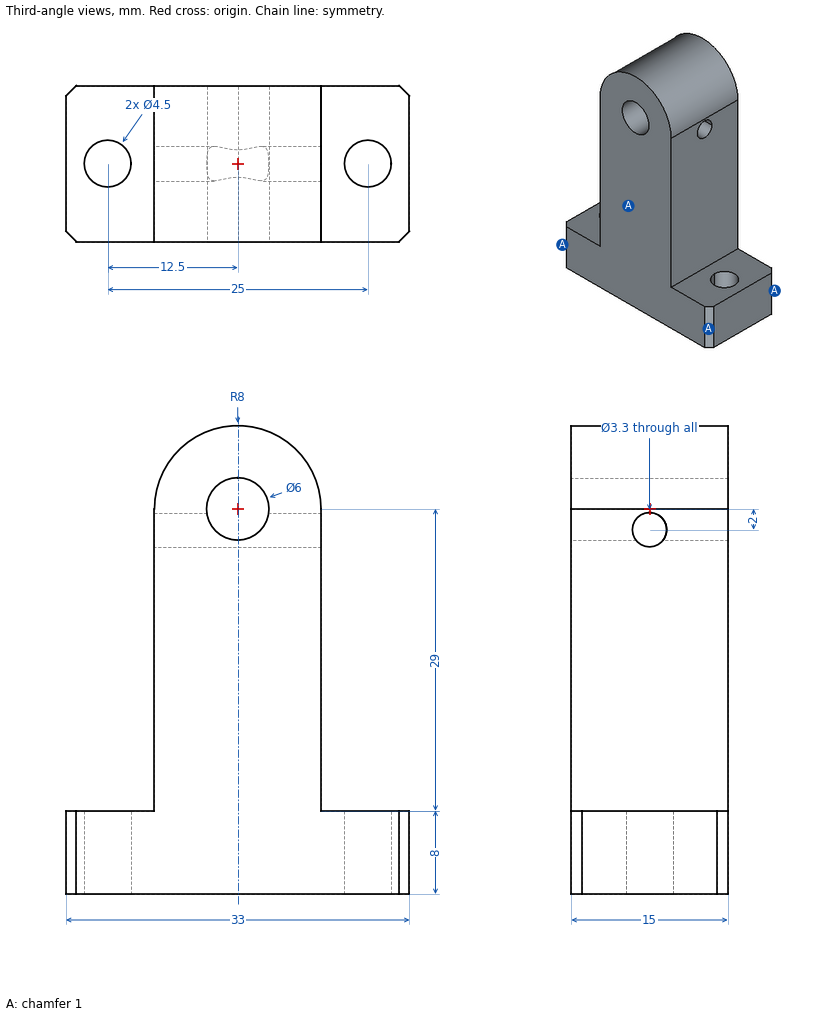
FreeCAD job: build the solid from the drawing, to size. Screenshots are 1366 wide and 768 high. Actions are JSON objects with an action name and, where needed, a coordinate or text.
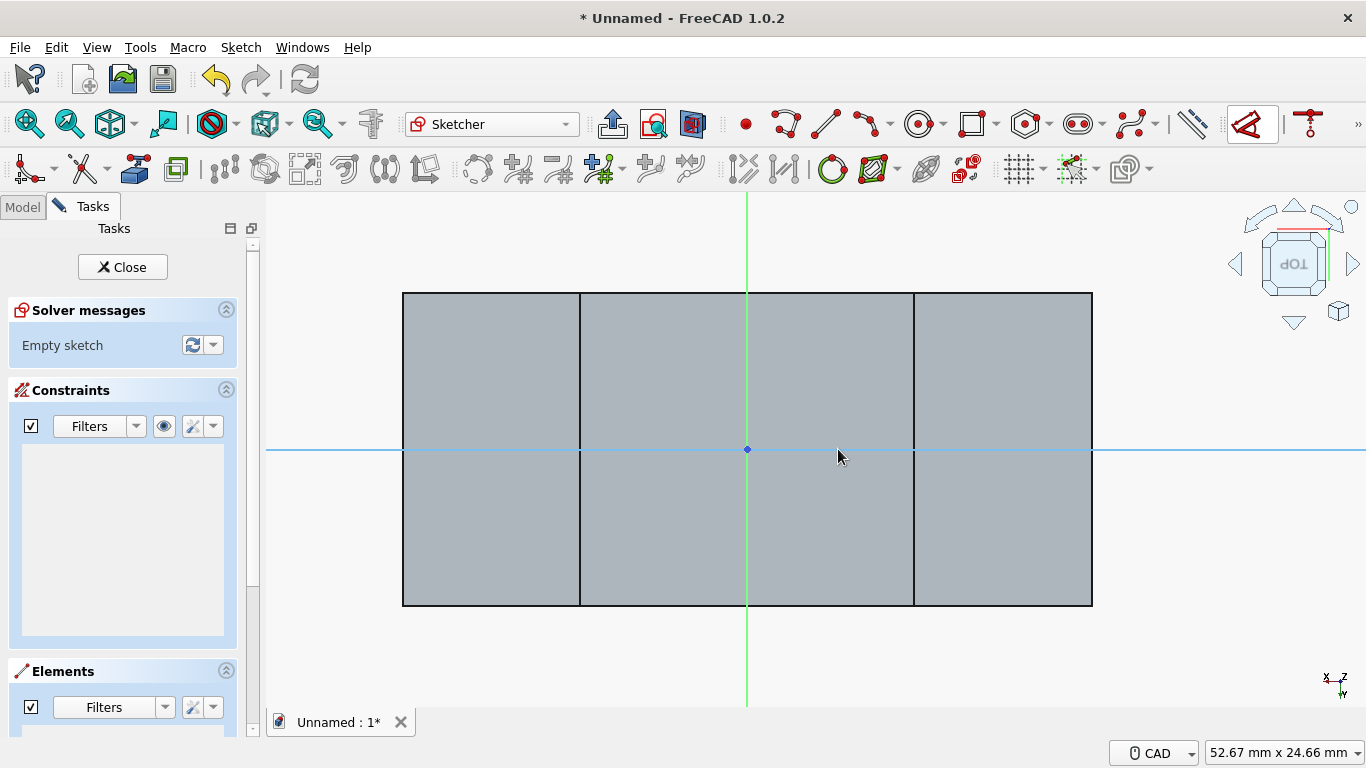
{"action": "key", "text": "g c"}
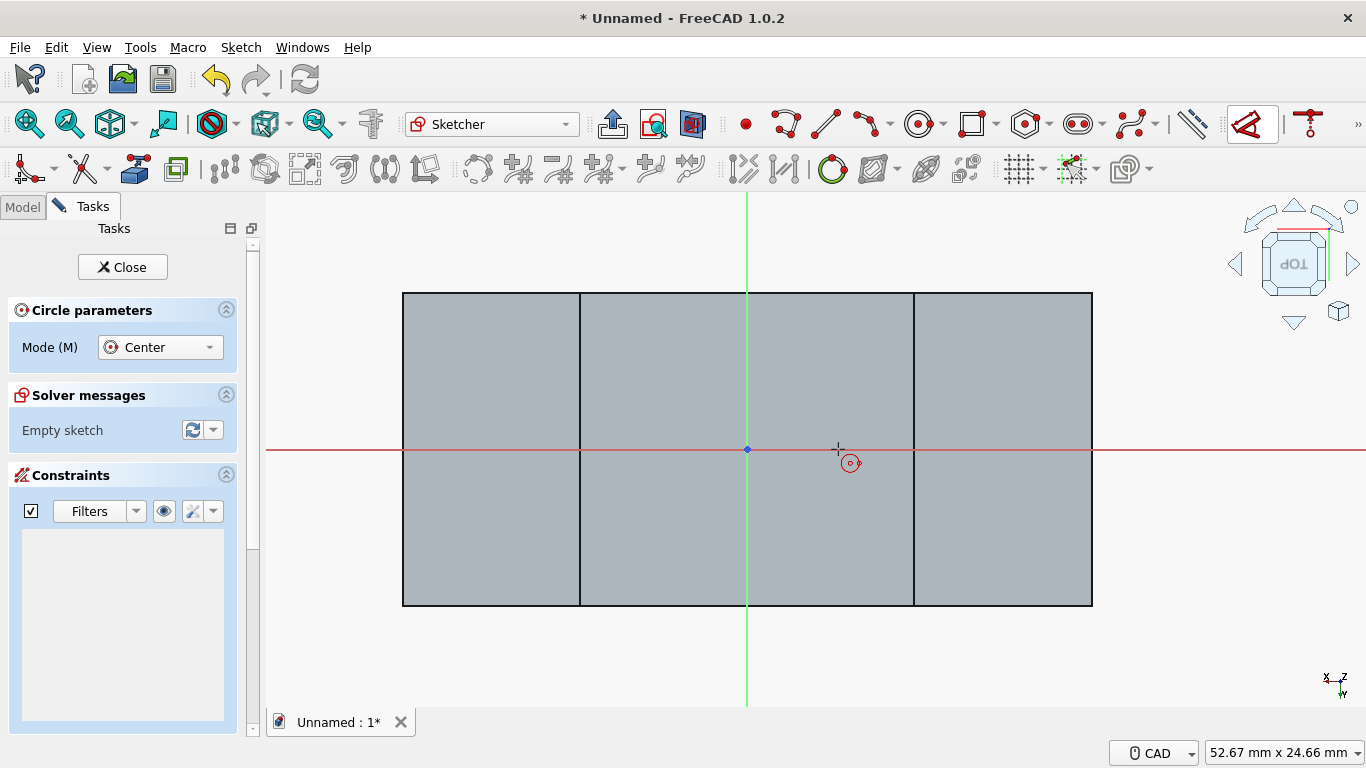
{"action": "left_click", "coordinate": [1008, 449]}
{"action": "mouse_move", "coordinate": [1041, 416]}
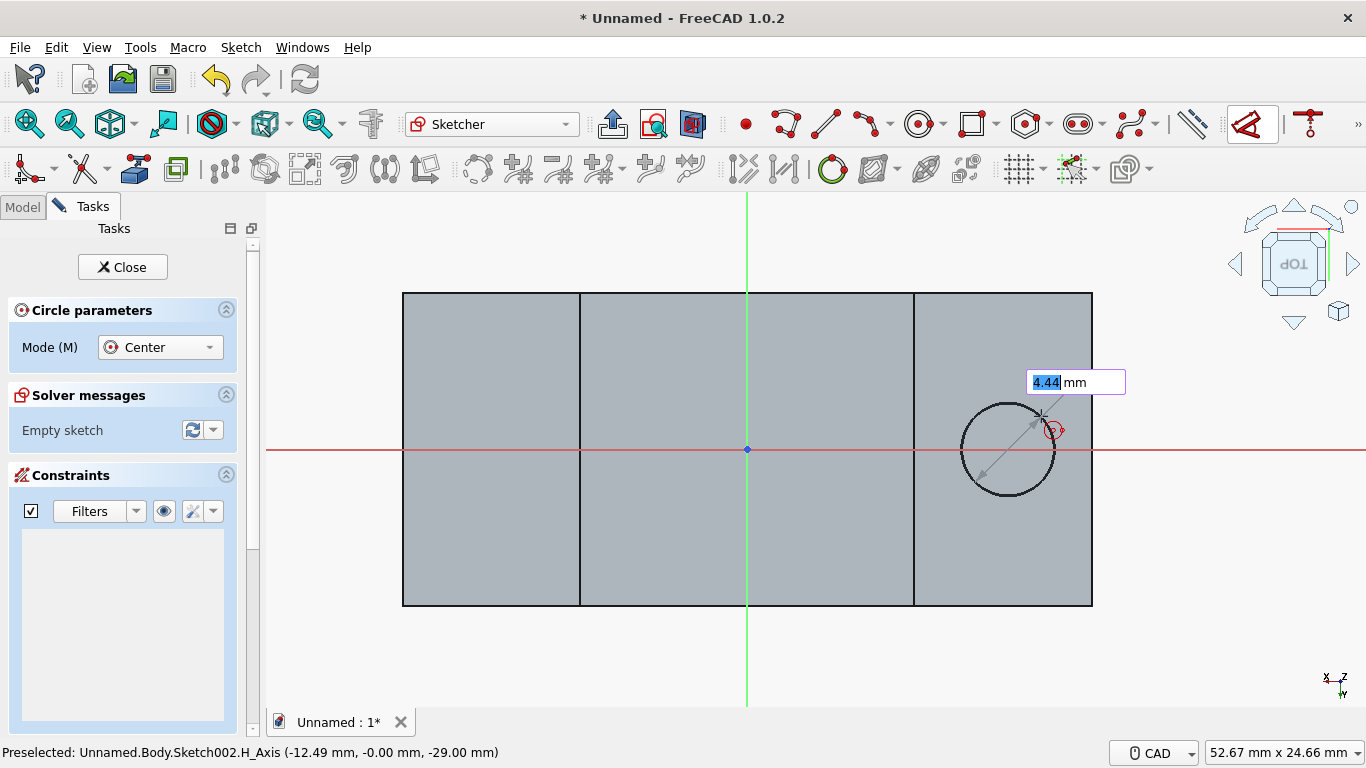
{"action": "type", "text": "4.5"}
{"action": "key", "text": "Return"}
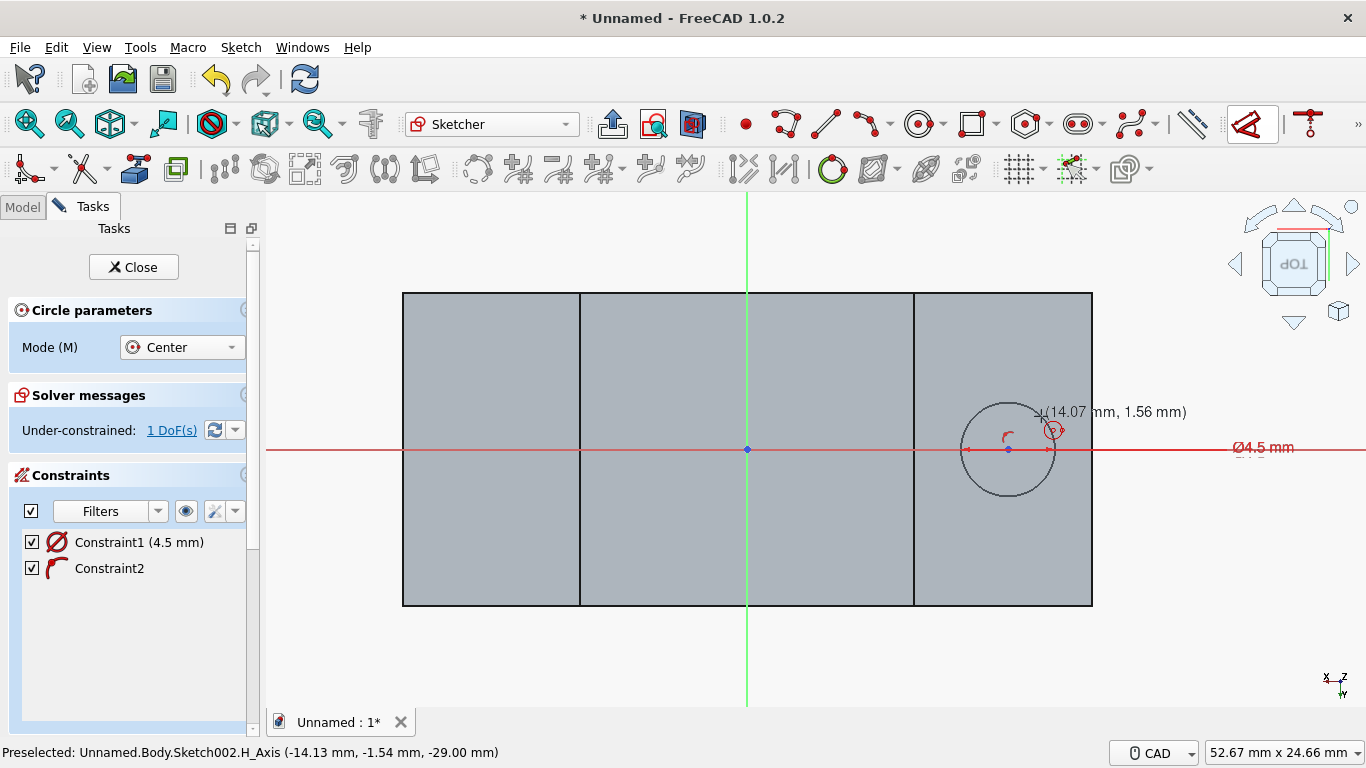
{"action": "left_click", "coordinate": [486, 449]}
{"action": "mouse_move", "coordinate": [519, 416]}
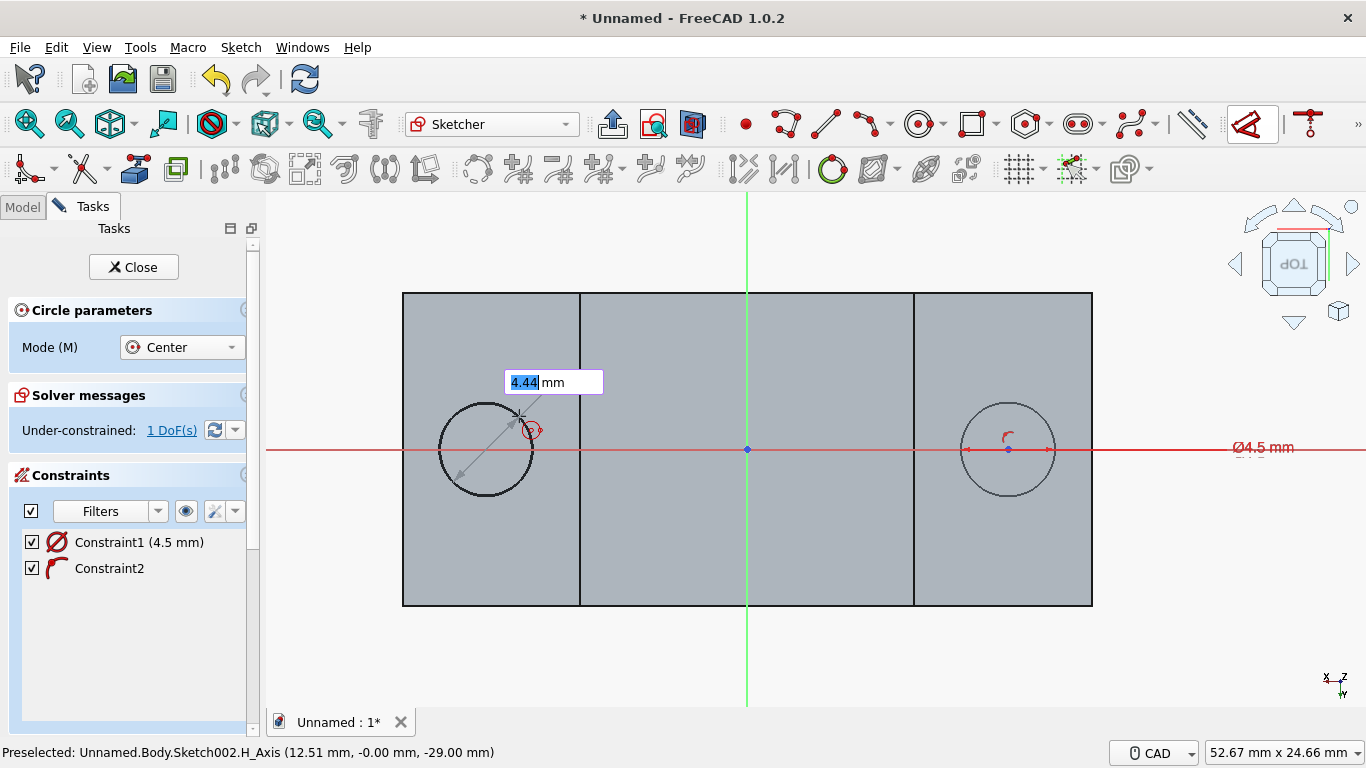
{"action": "type", "text": "4.5"}
{"action": "key", "text": "Return"}
{"action": "key", "text": "Escape"}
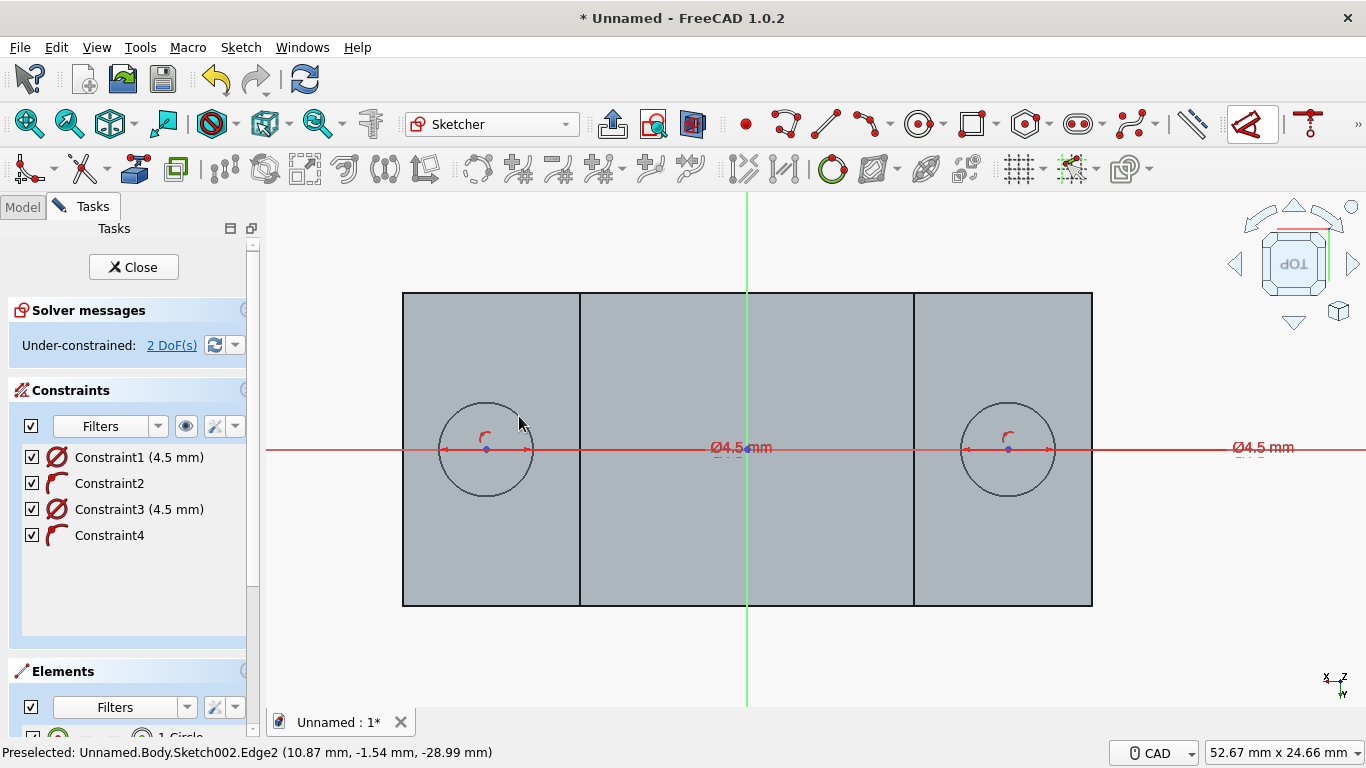
{"action": "left_click", "coordinate": [1246, 124]}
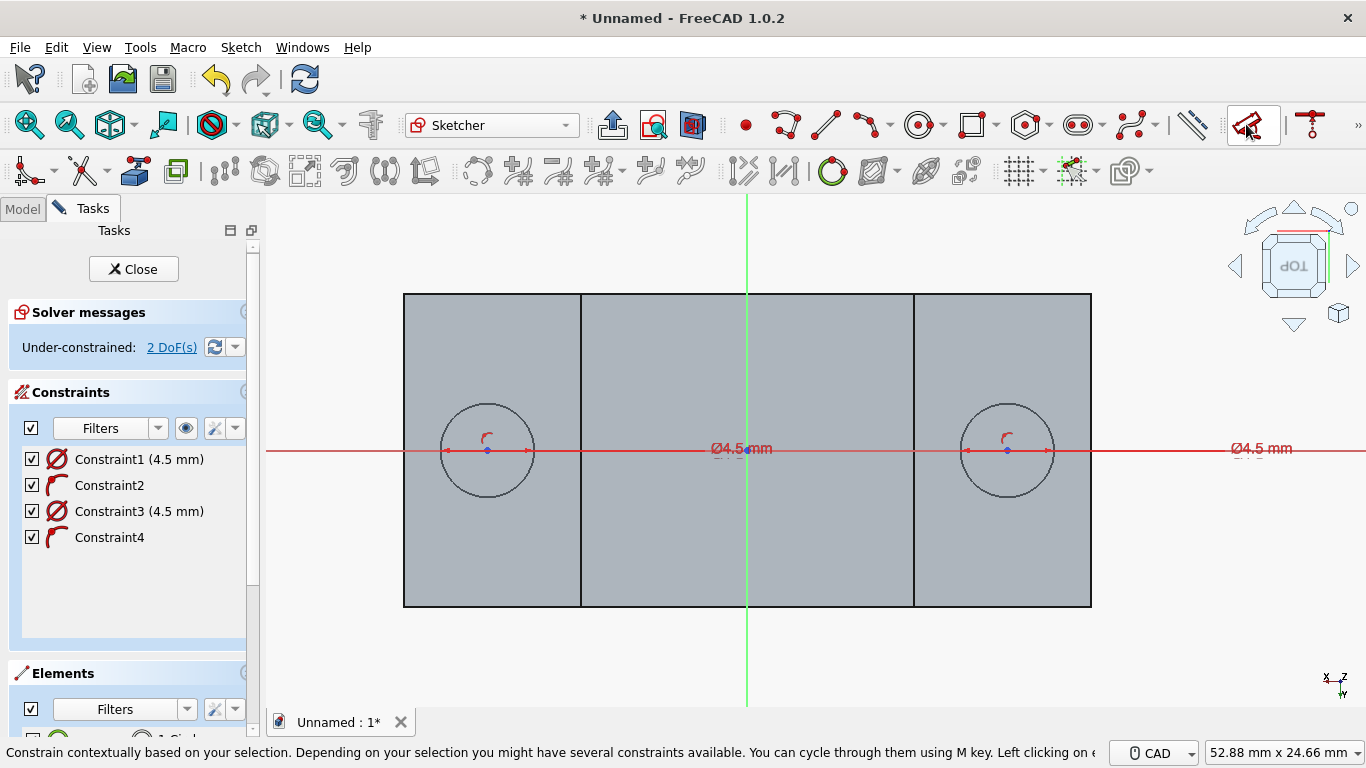
{"action": "left_click", "coordinate": [1007, 450]}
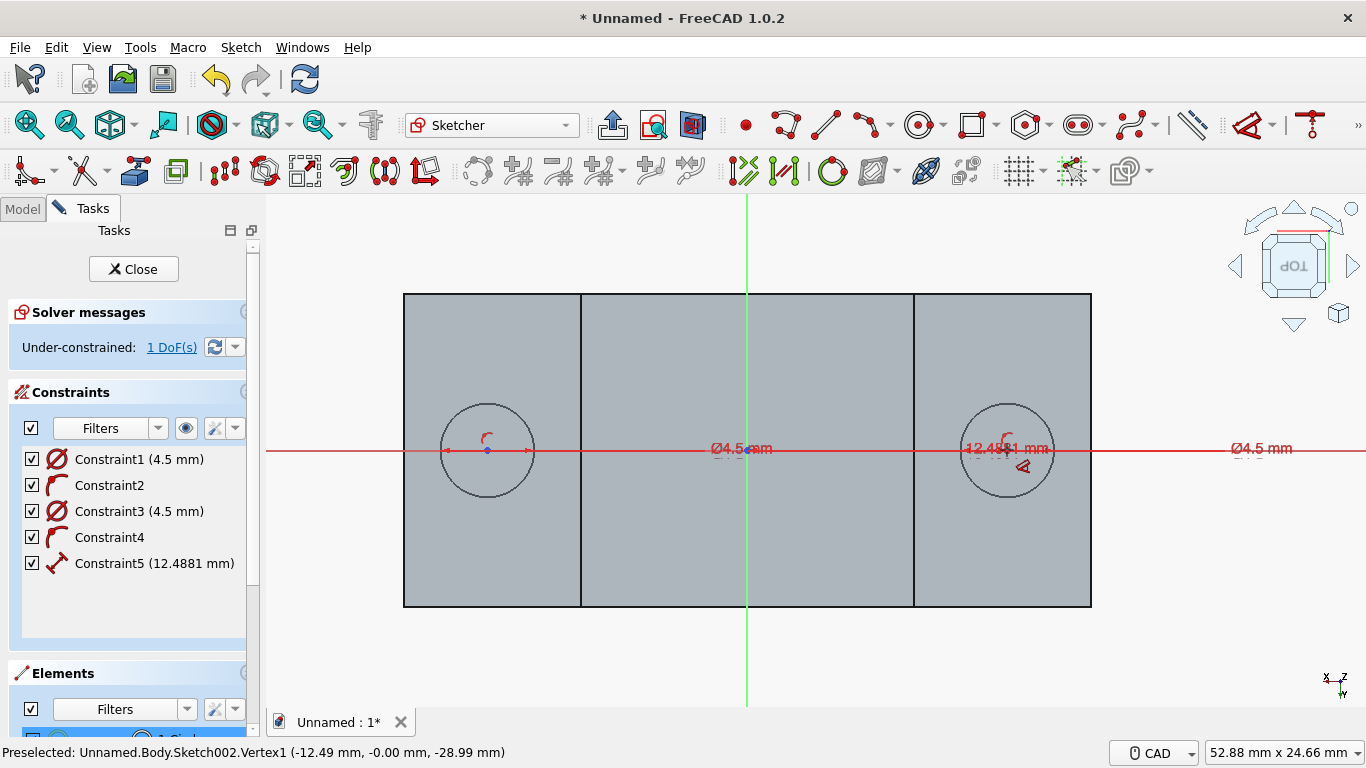
{"action": "left_click", "coordinate": [487, 450]}
{"action": "left_click", "coordinate": [628, 484]}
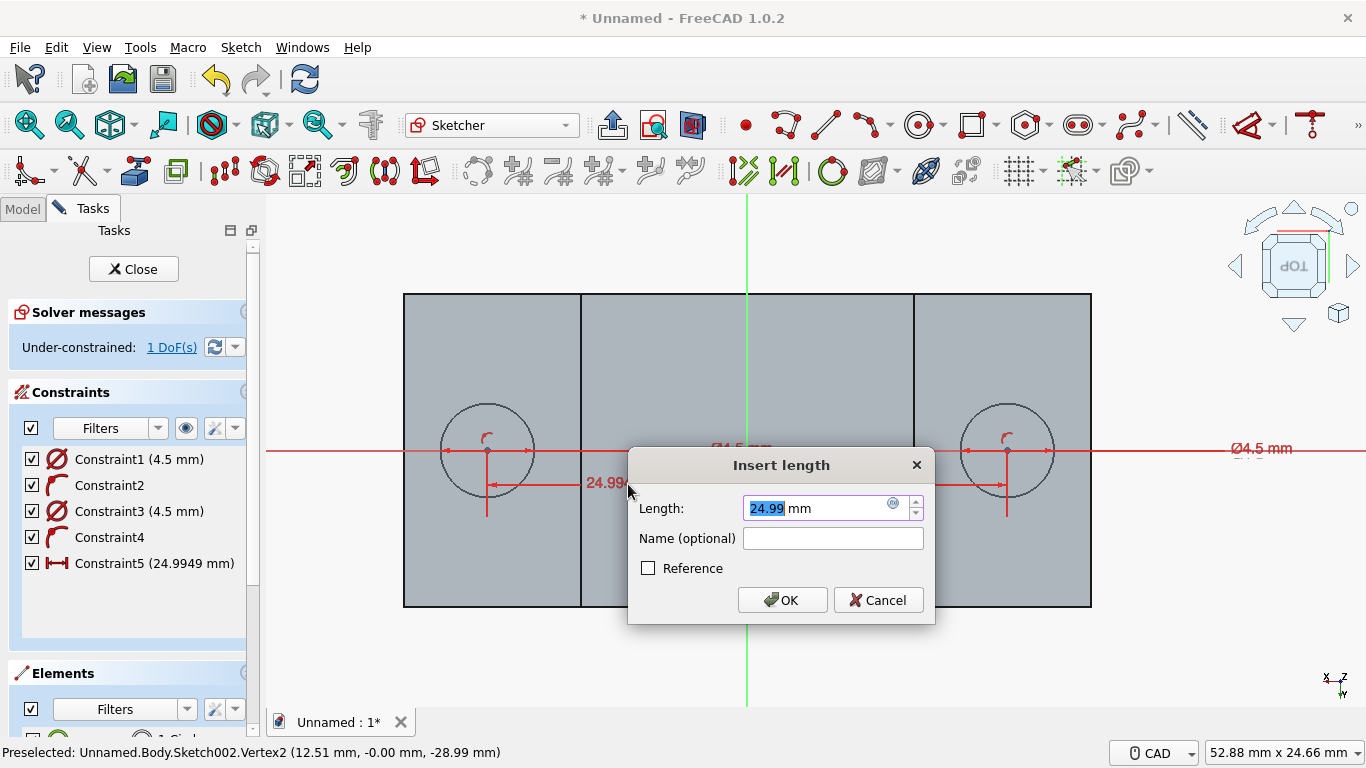
{"action": "type", "text": "25"}
{"action": "key", "text": "Return"}